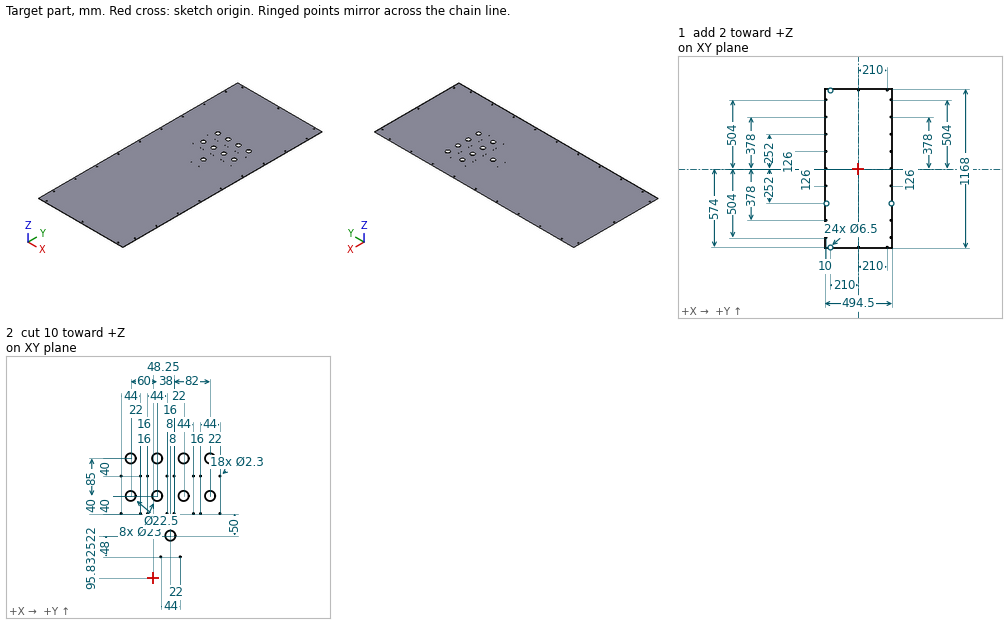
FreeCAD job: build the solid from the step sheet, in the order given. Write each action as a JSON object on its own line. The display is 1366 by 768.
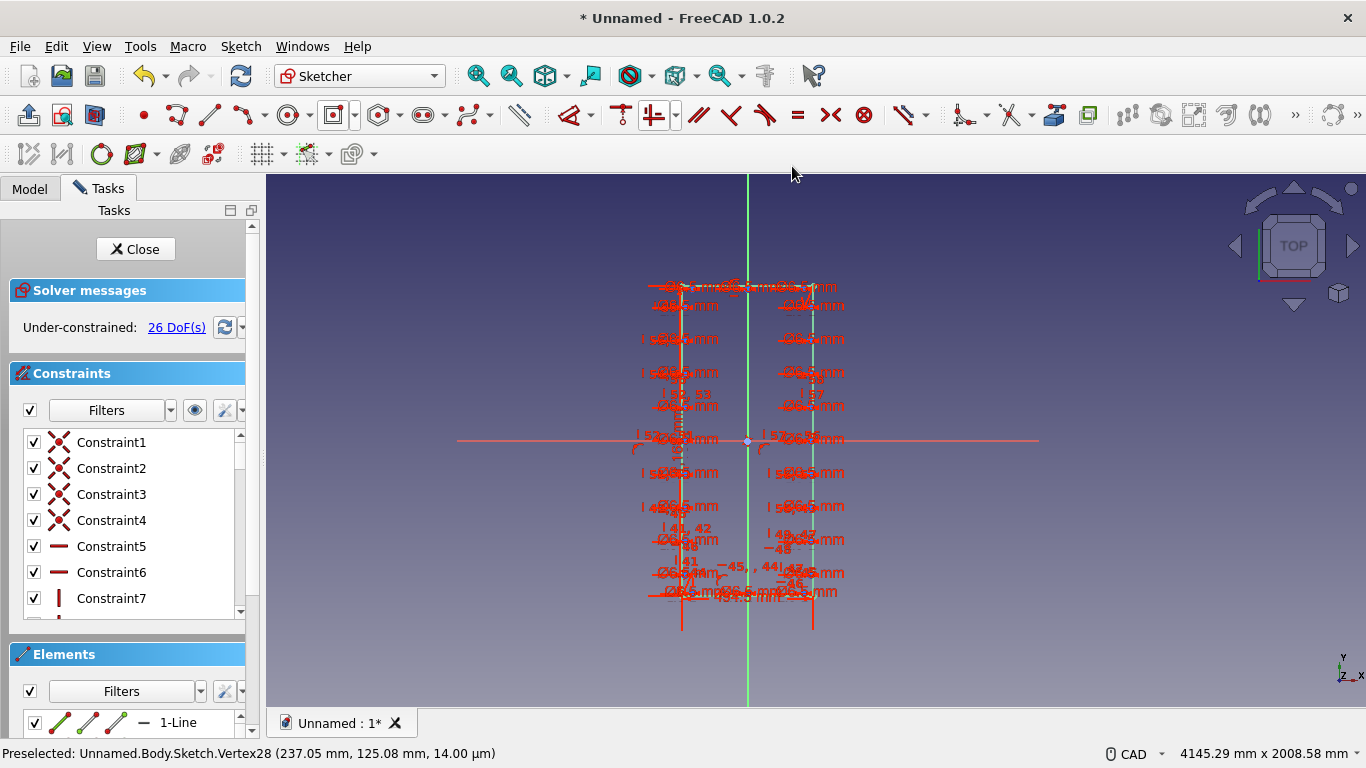
{"action": "left_click", "coordinate": [811, 408]}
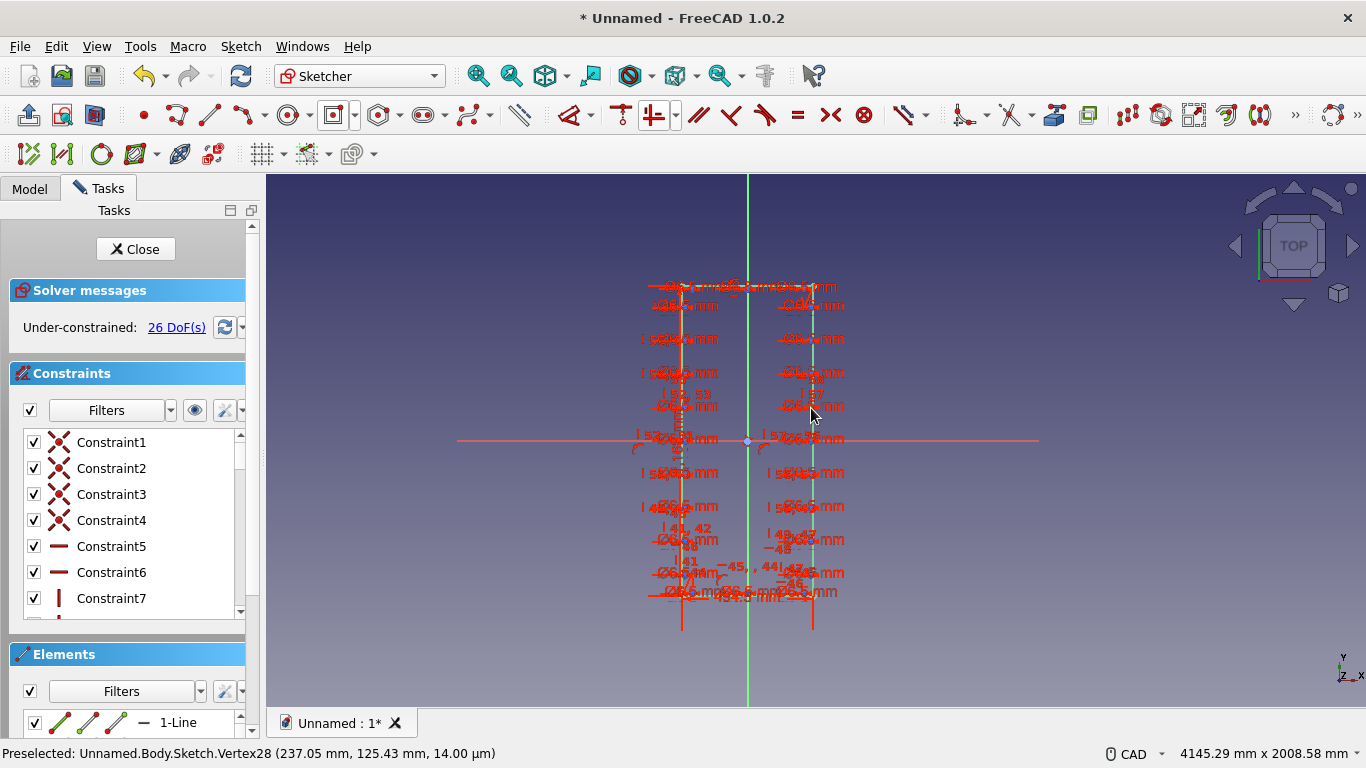
{"action": "scroll", "coordinate": [811, 374], "scroll_direction": "up", "scroll_amount": 4}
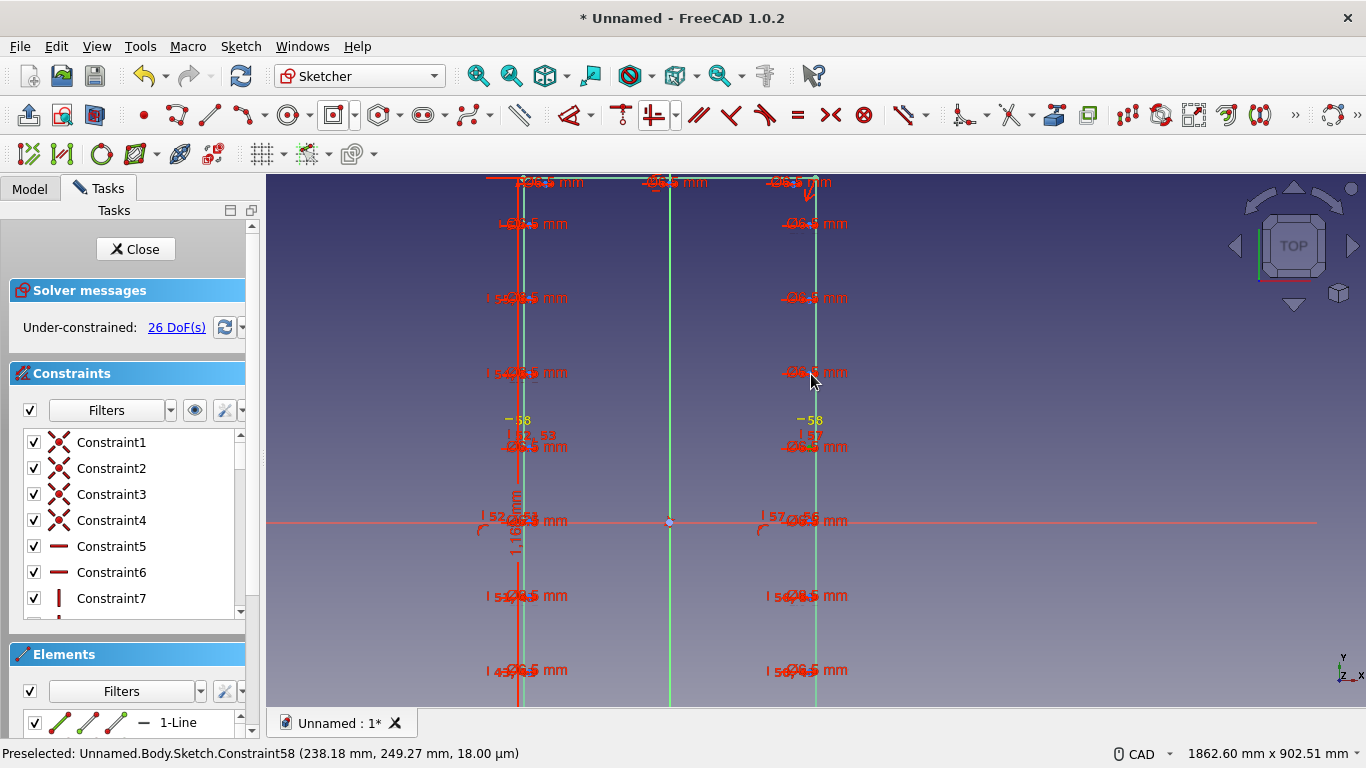
{"action": "left_click", "coordinate": [810, 374]}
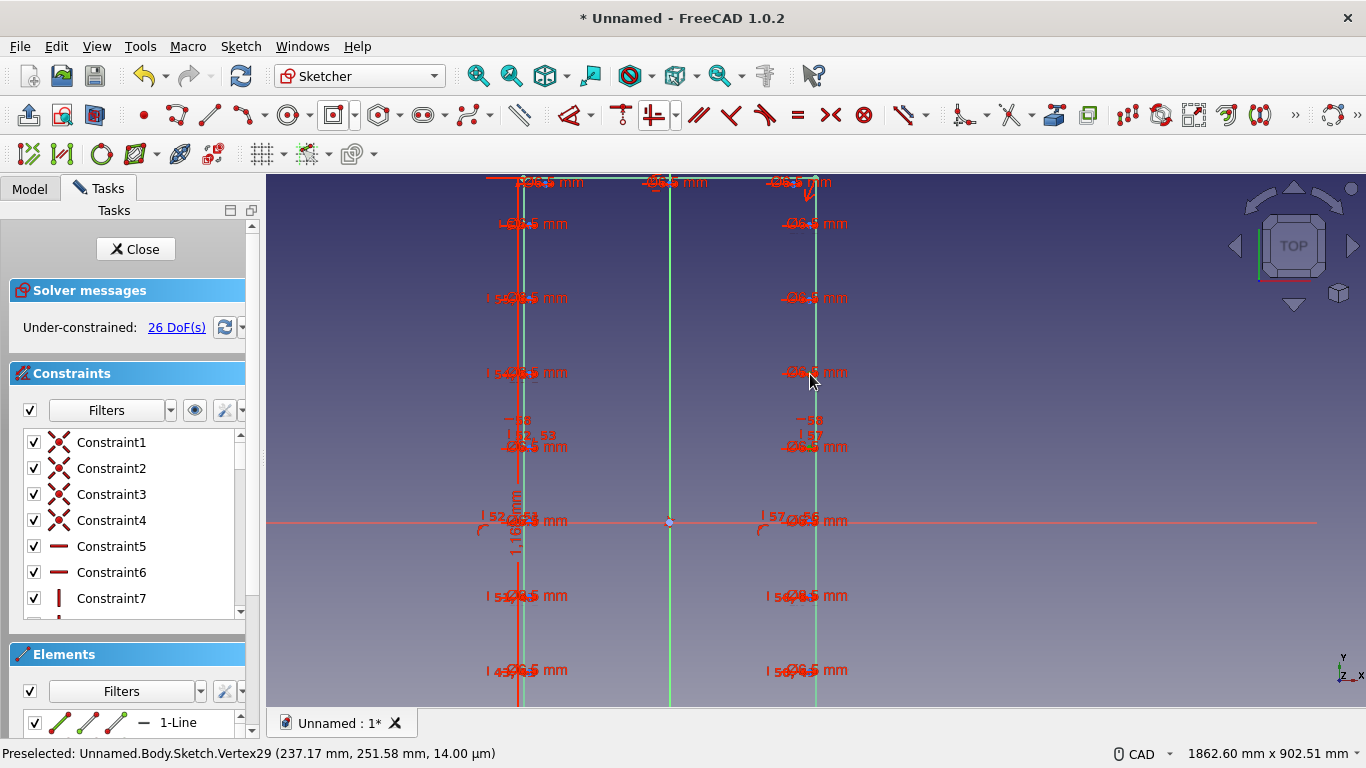
{"action": "left_click", "coordinate": [676, 116]}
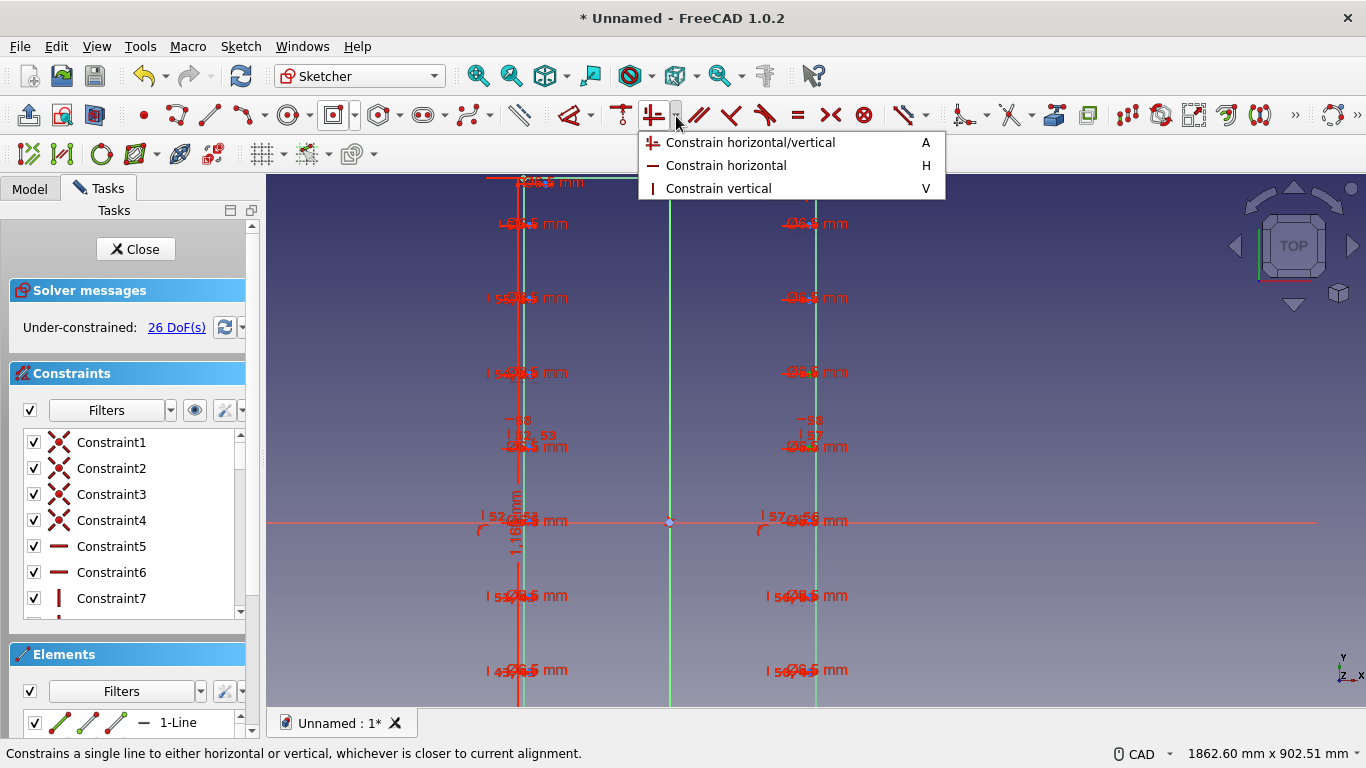
{"action": "left_click", "coordinate": [792, 188]}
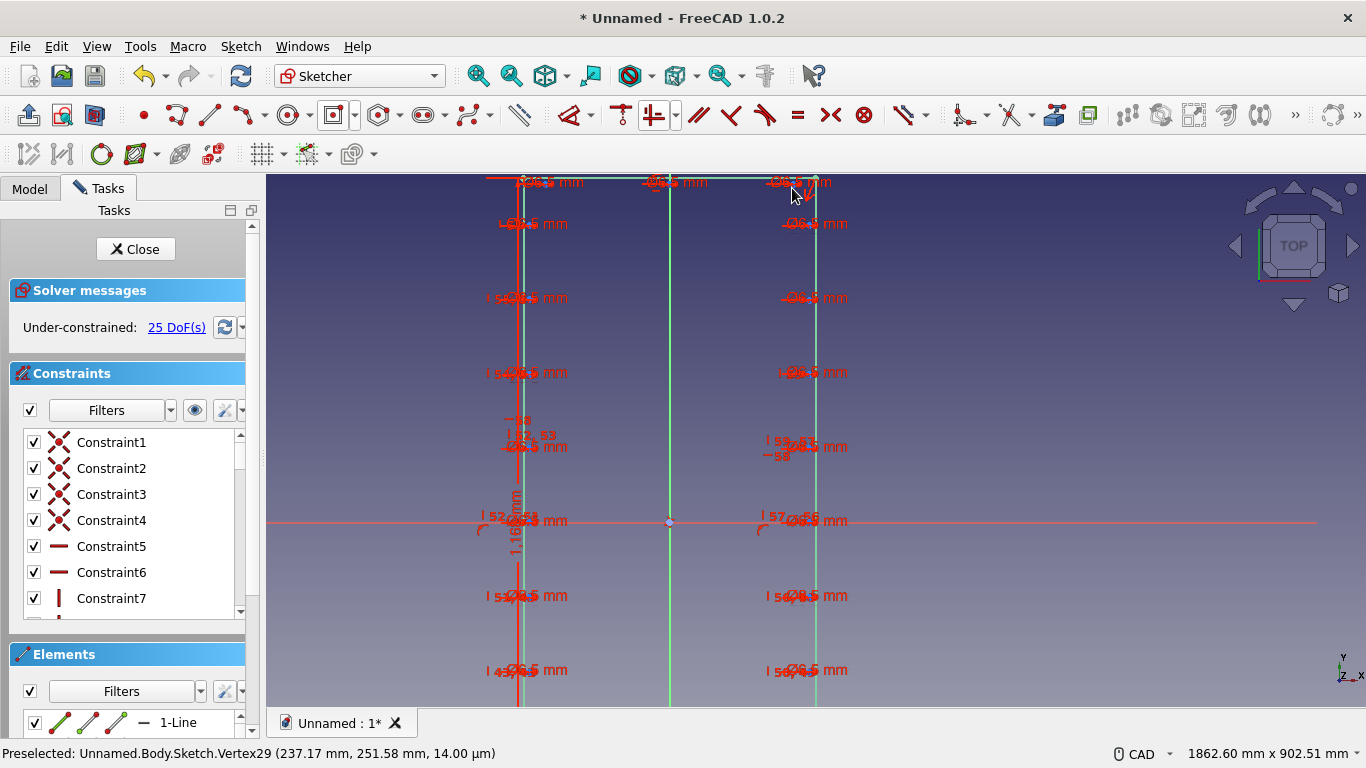
{"action": "left_click", "coordinate": [530, 375]}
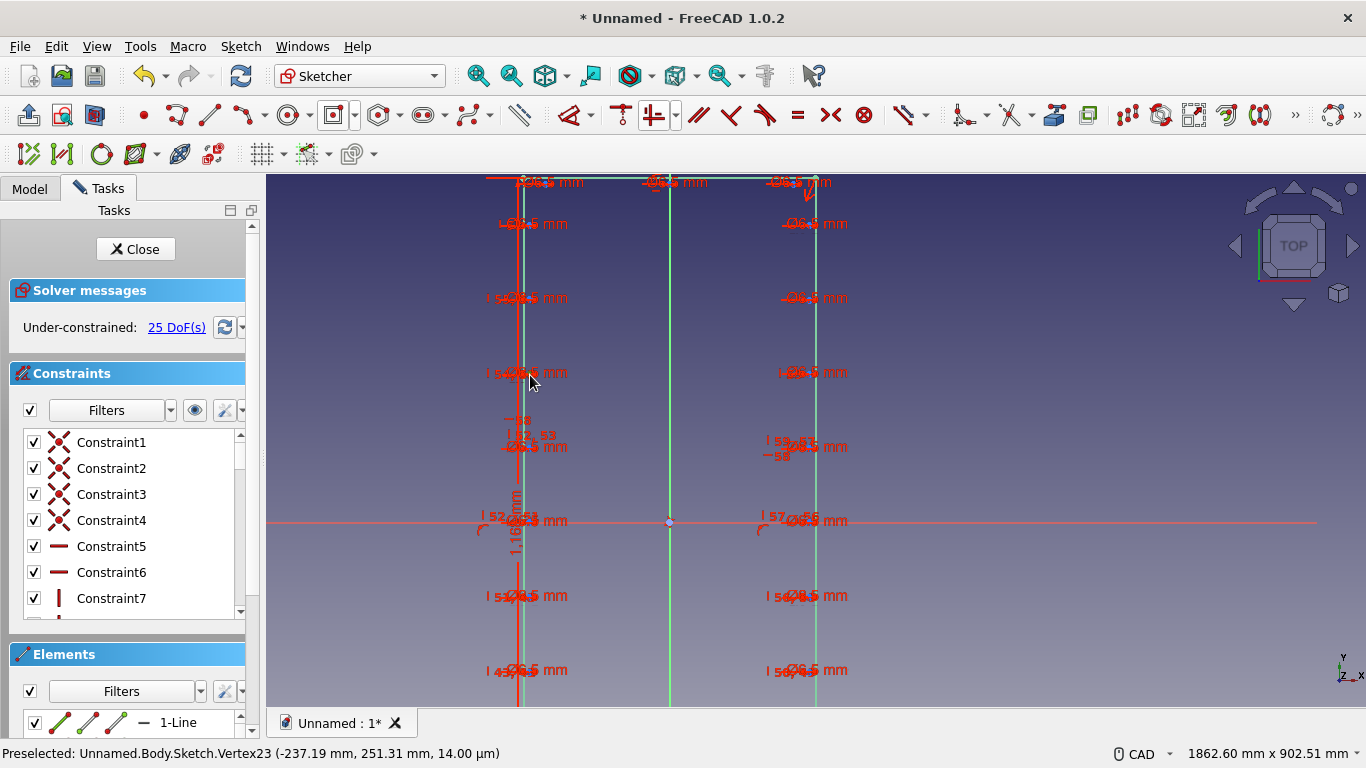
{"action": "left_click", "coordinate": [810, 374]}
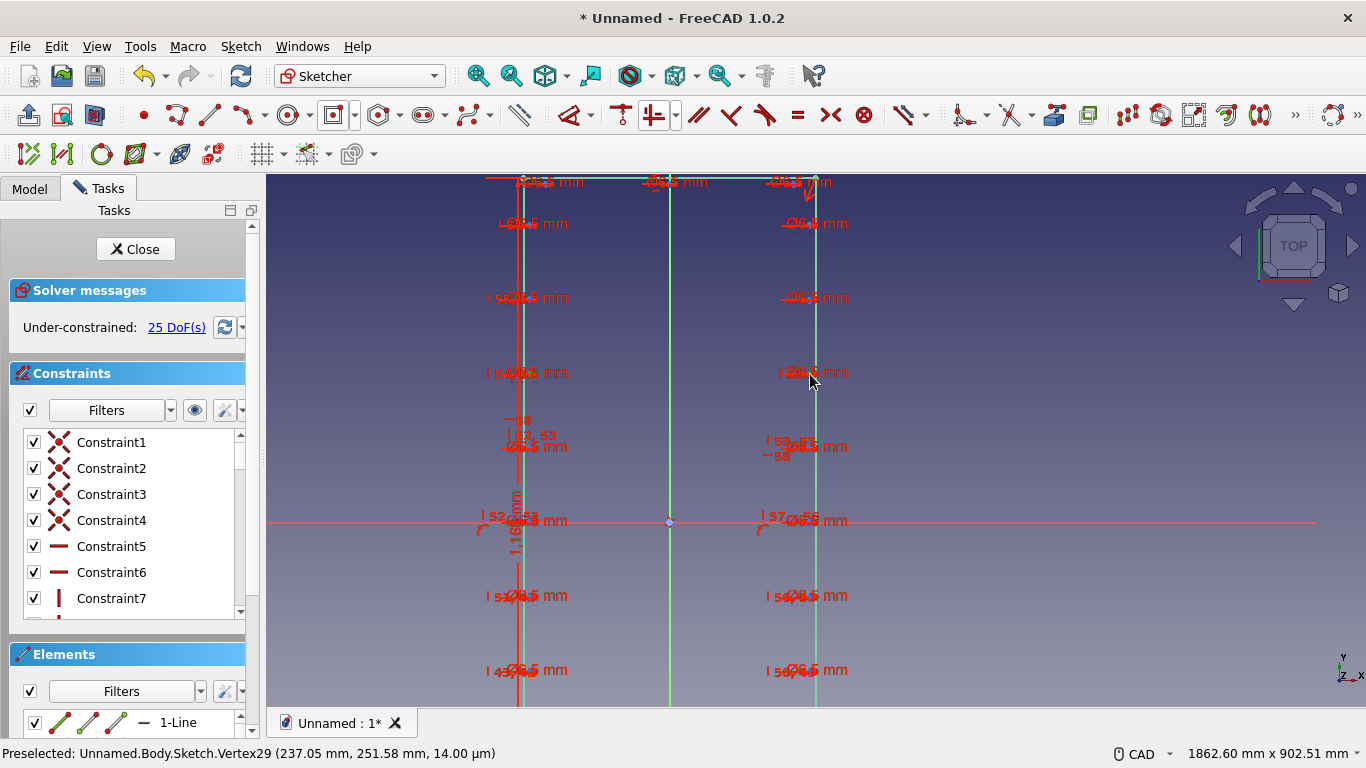
{"action": "key", "text": "h"}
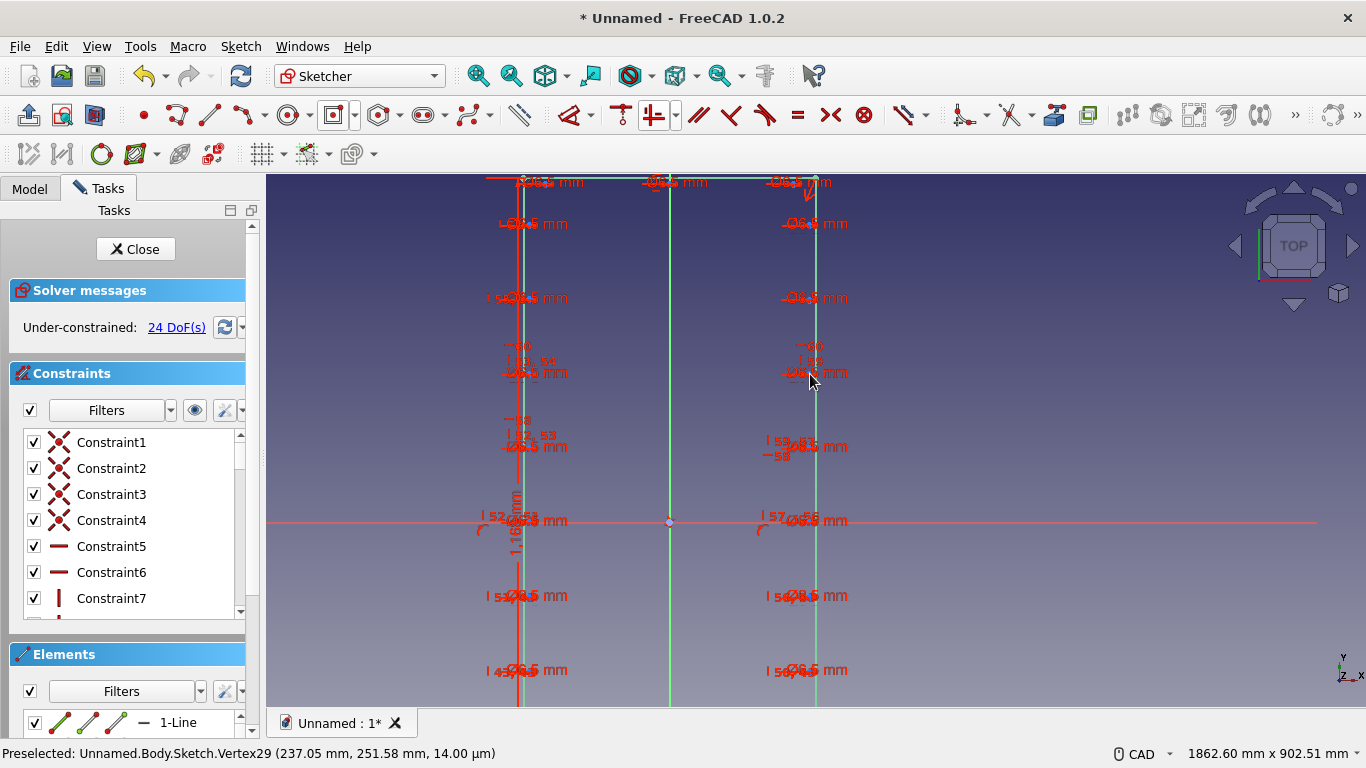
{"action": "scroll", "coordinate": [811, 373], "scroll_direction": "down", "scroll_amount": 4}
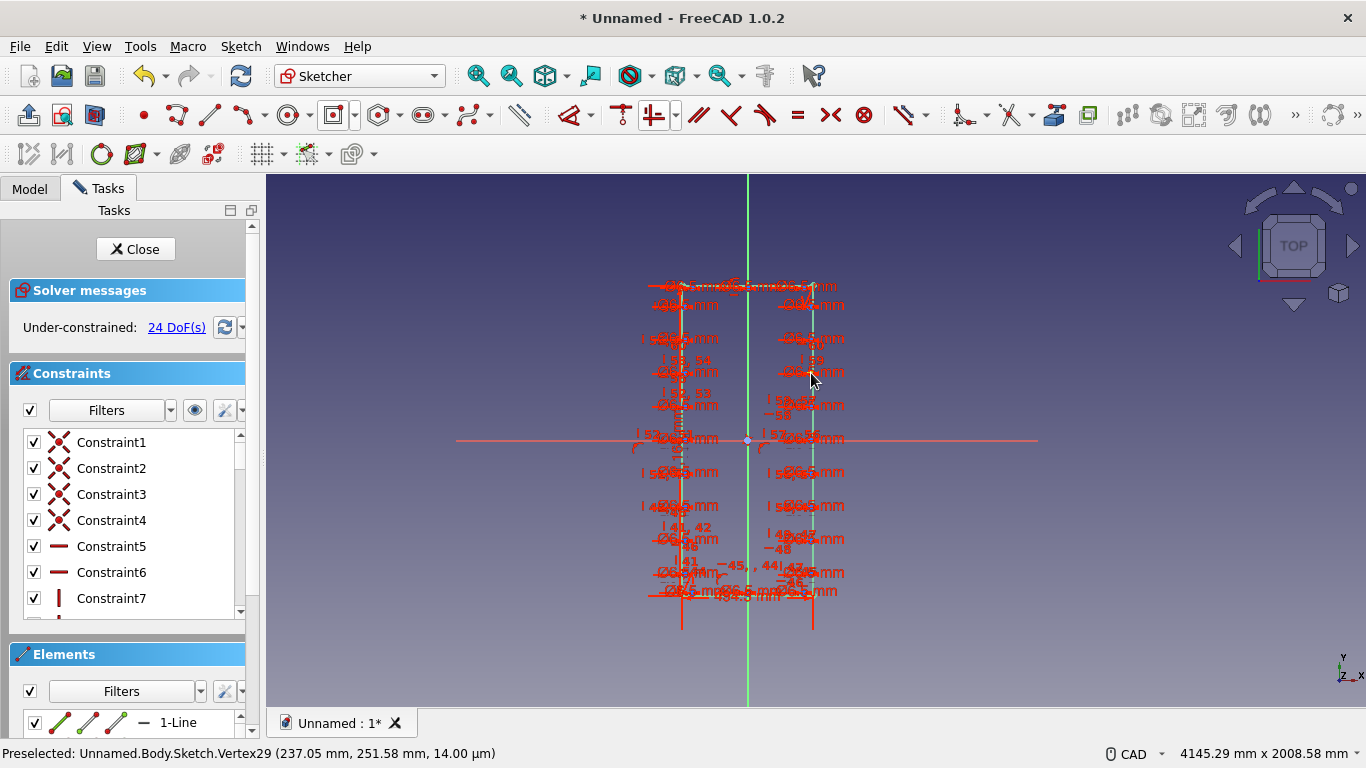
{"action": "left_click", "coordinate": [692, 288]}